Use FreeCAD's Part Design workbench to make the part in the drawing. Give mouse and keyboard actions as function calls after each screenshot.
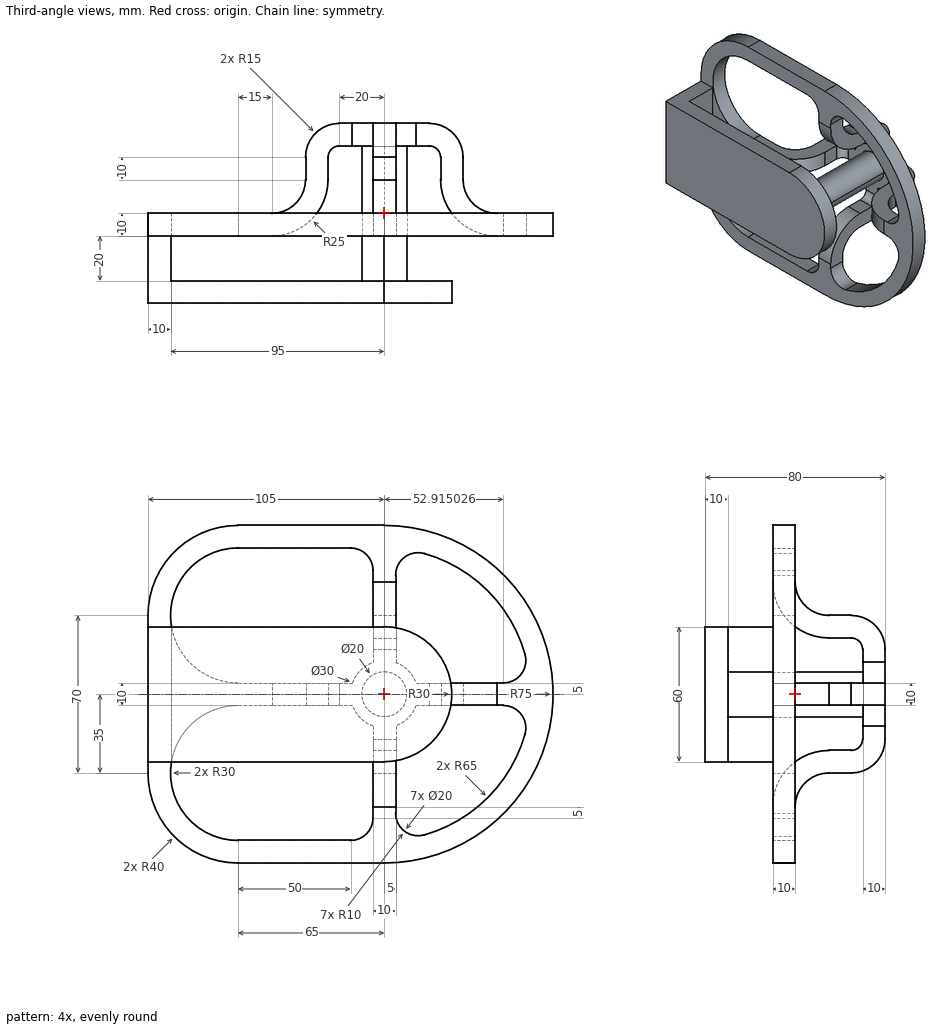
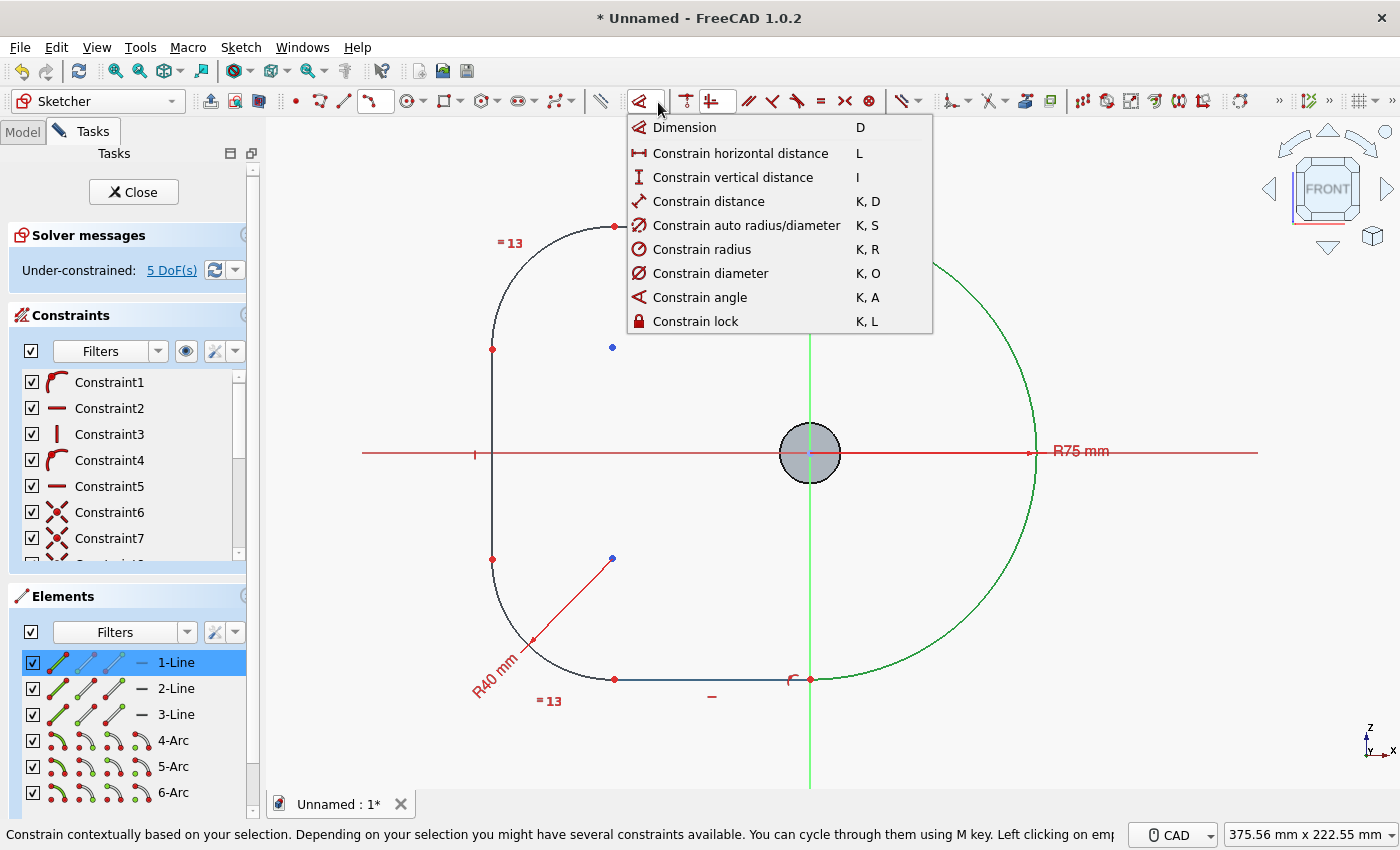
click(780, 153)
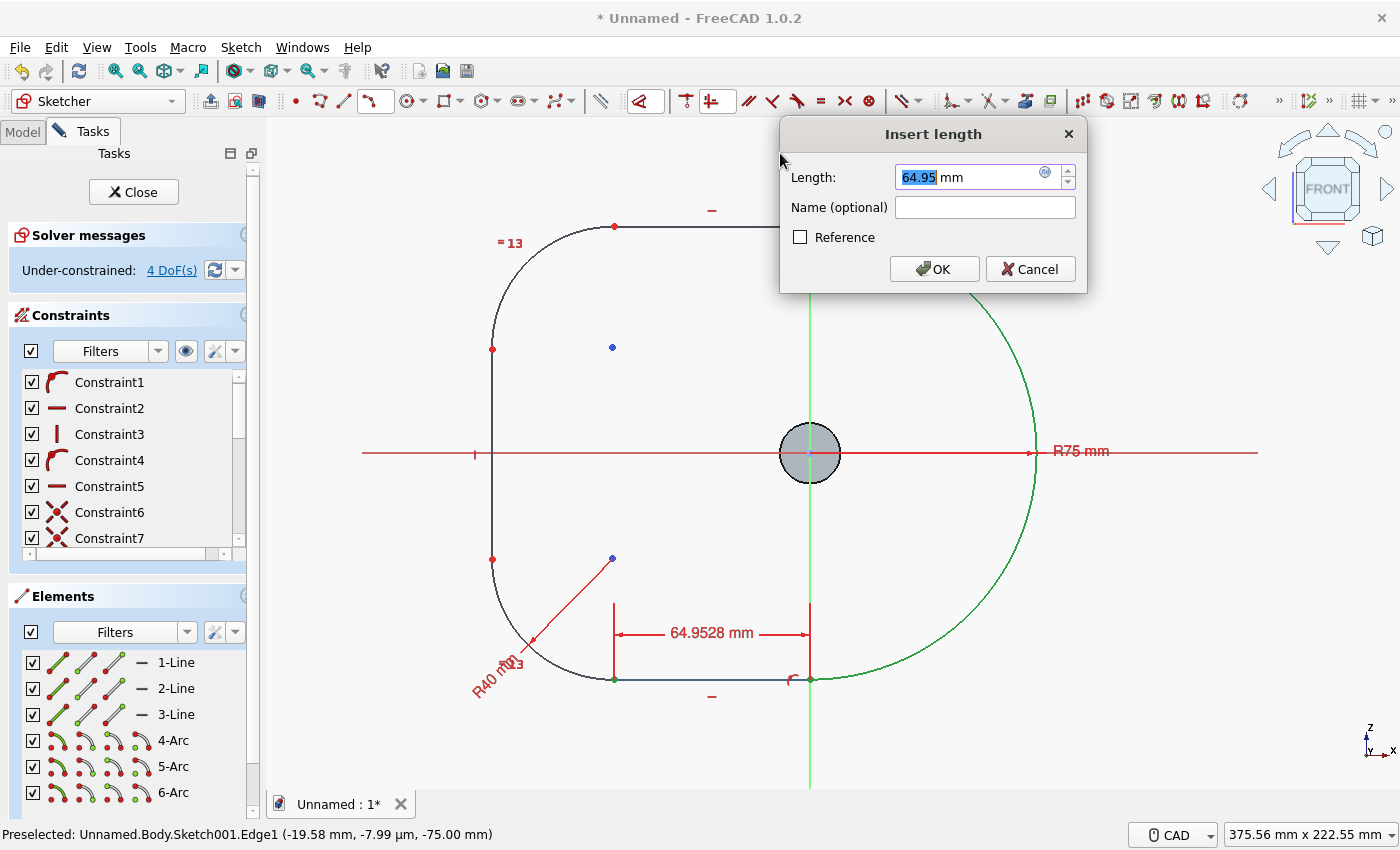
text(65)
key(Return)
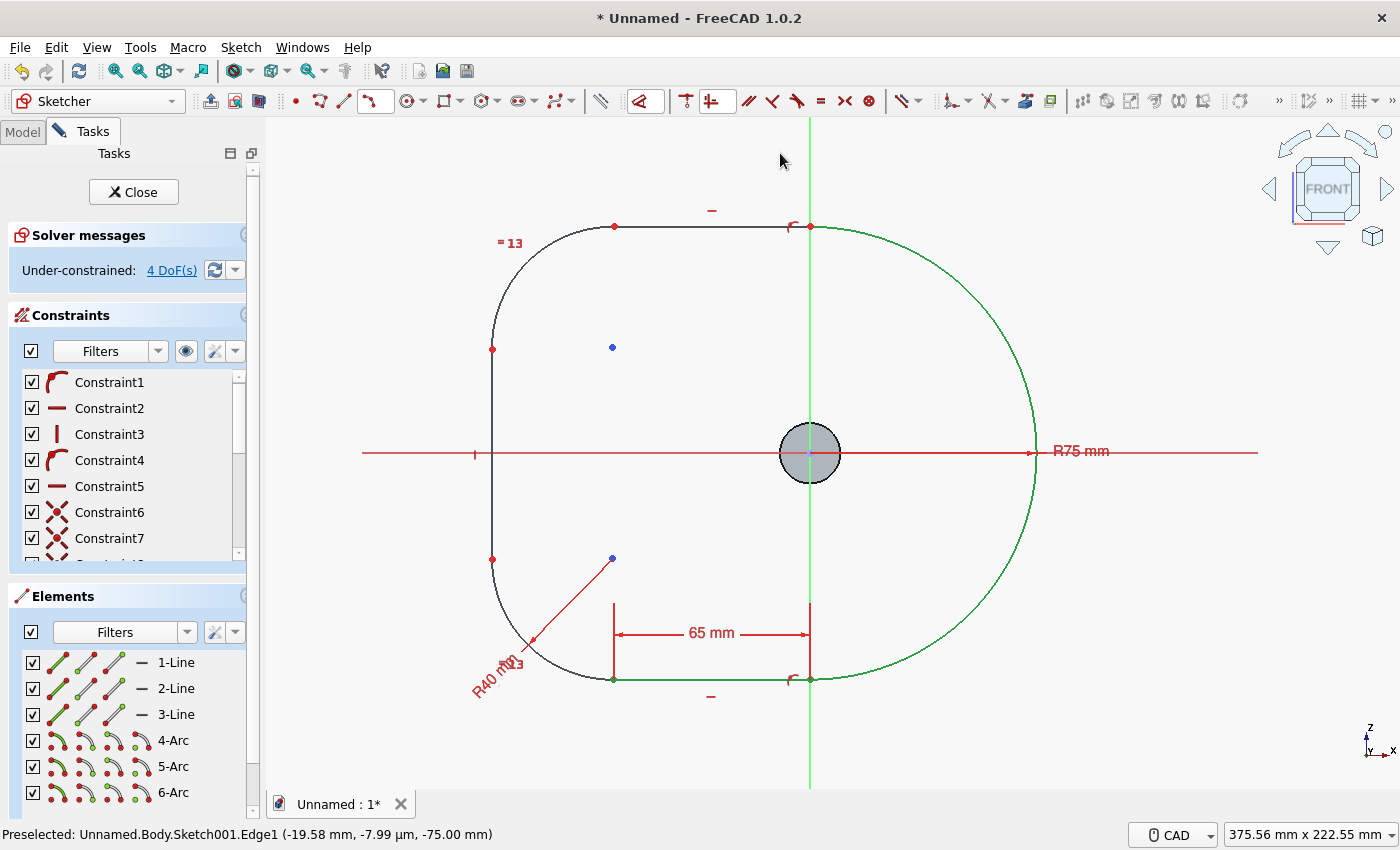
click(492, 497)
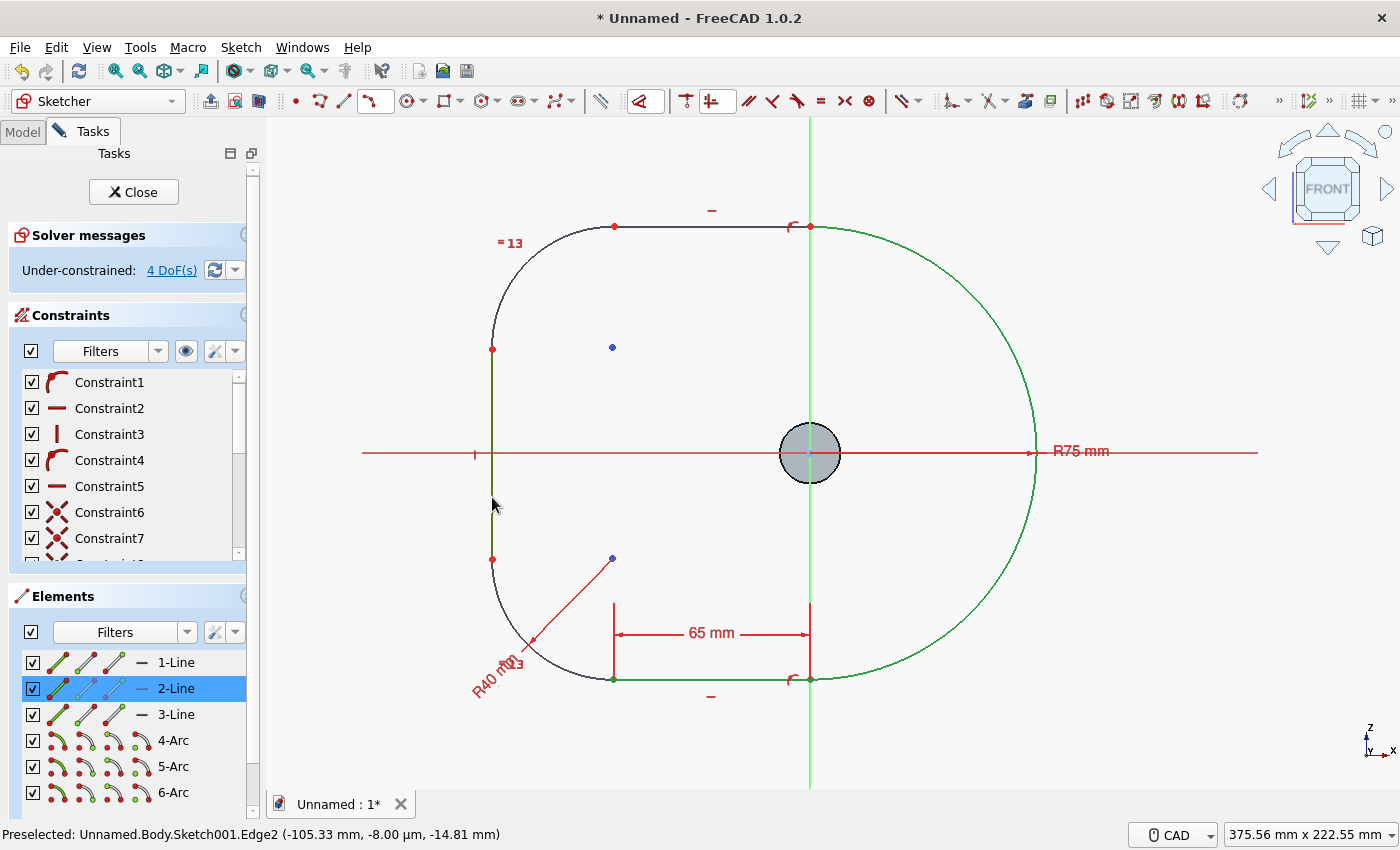
click(658, 102)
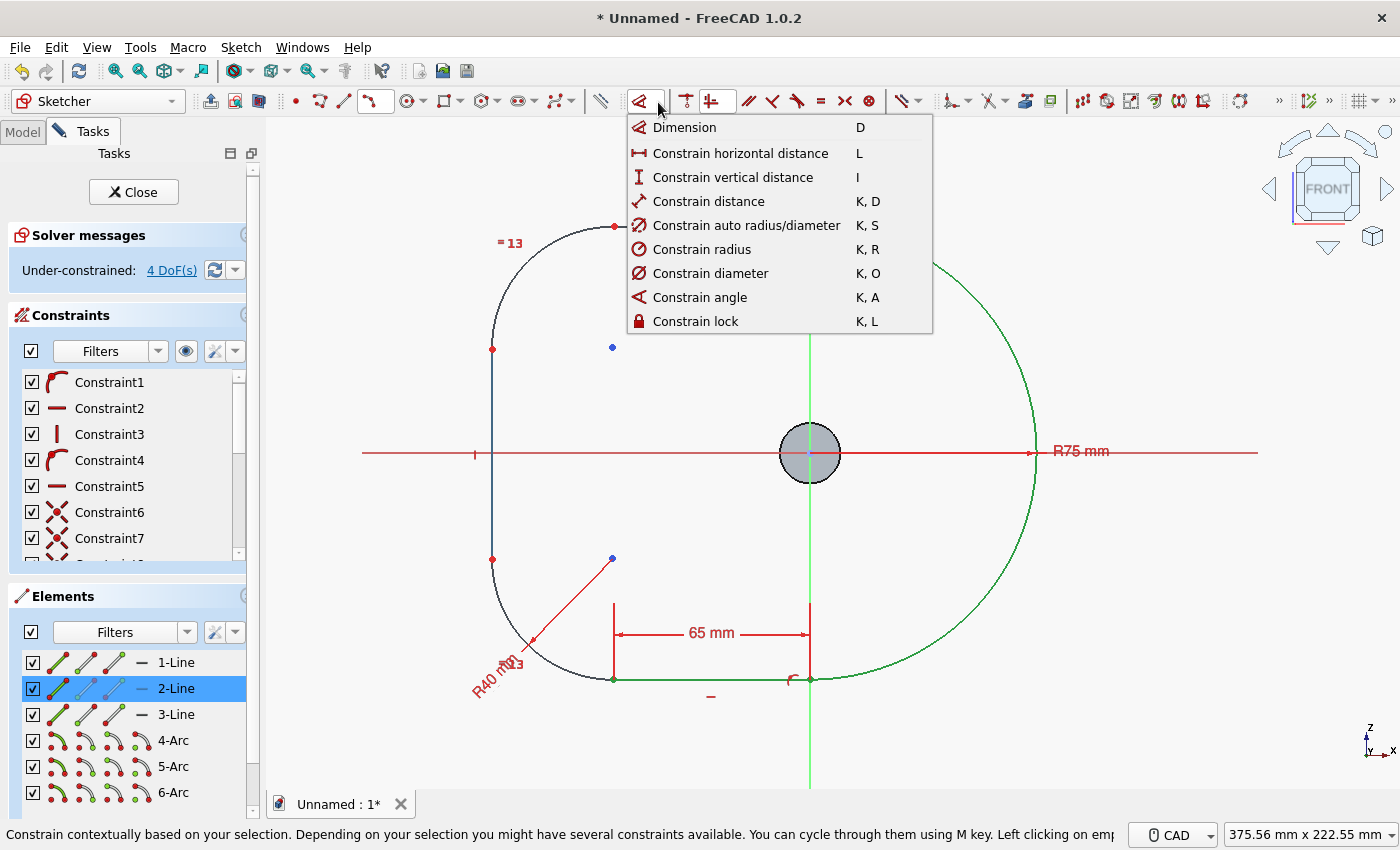
click(780, 177)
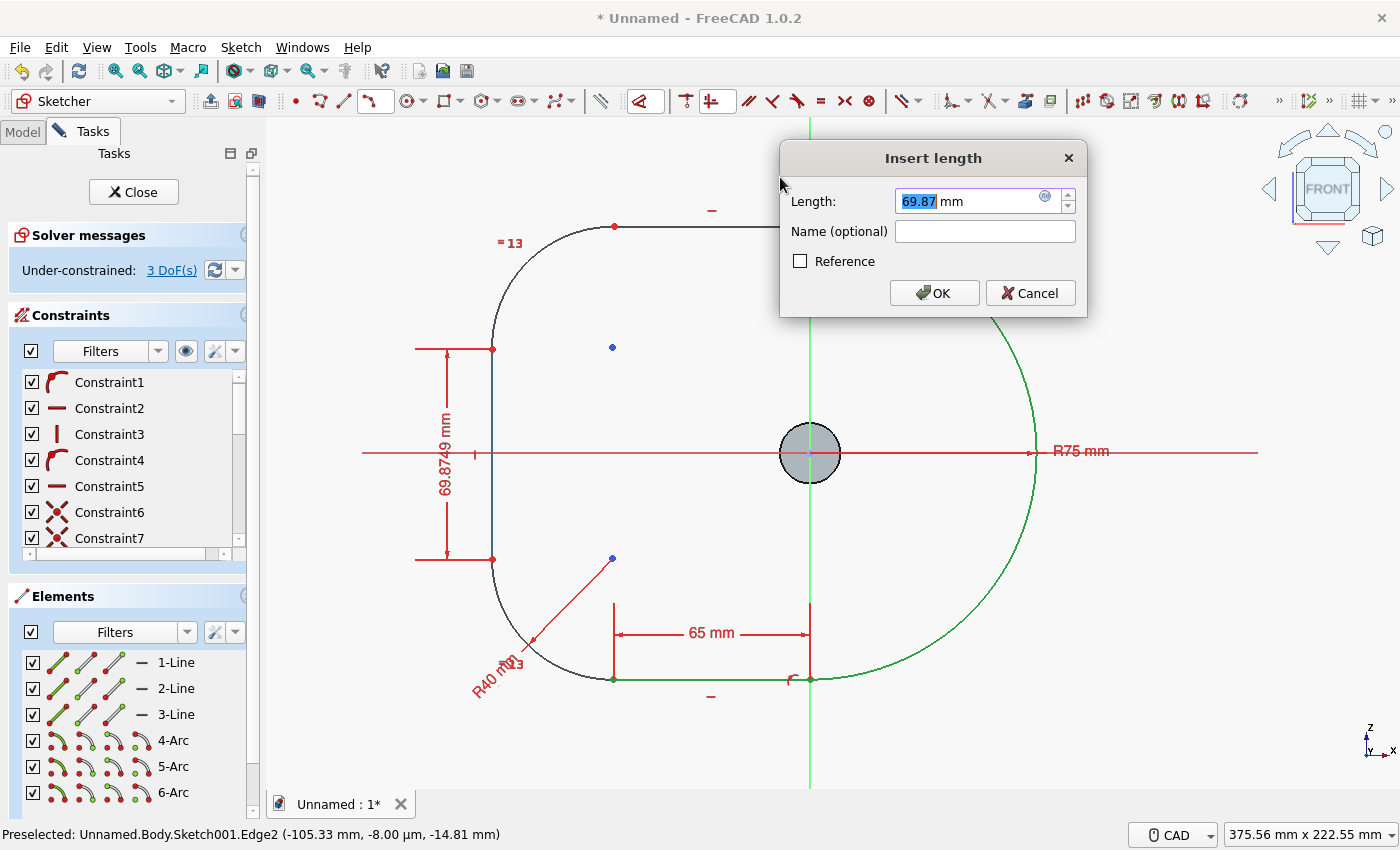
text(70)
key(Return)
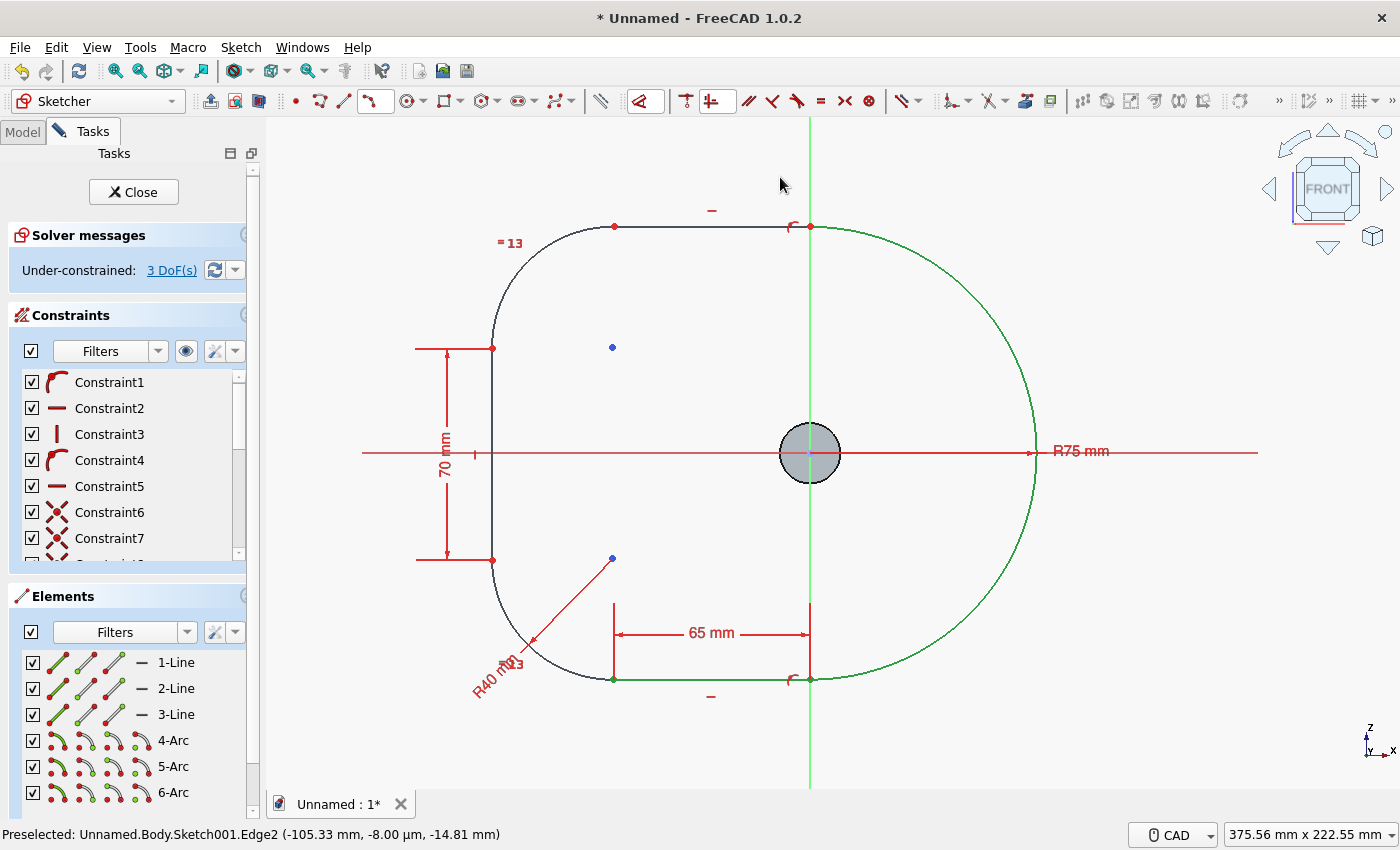
click(673, 227)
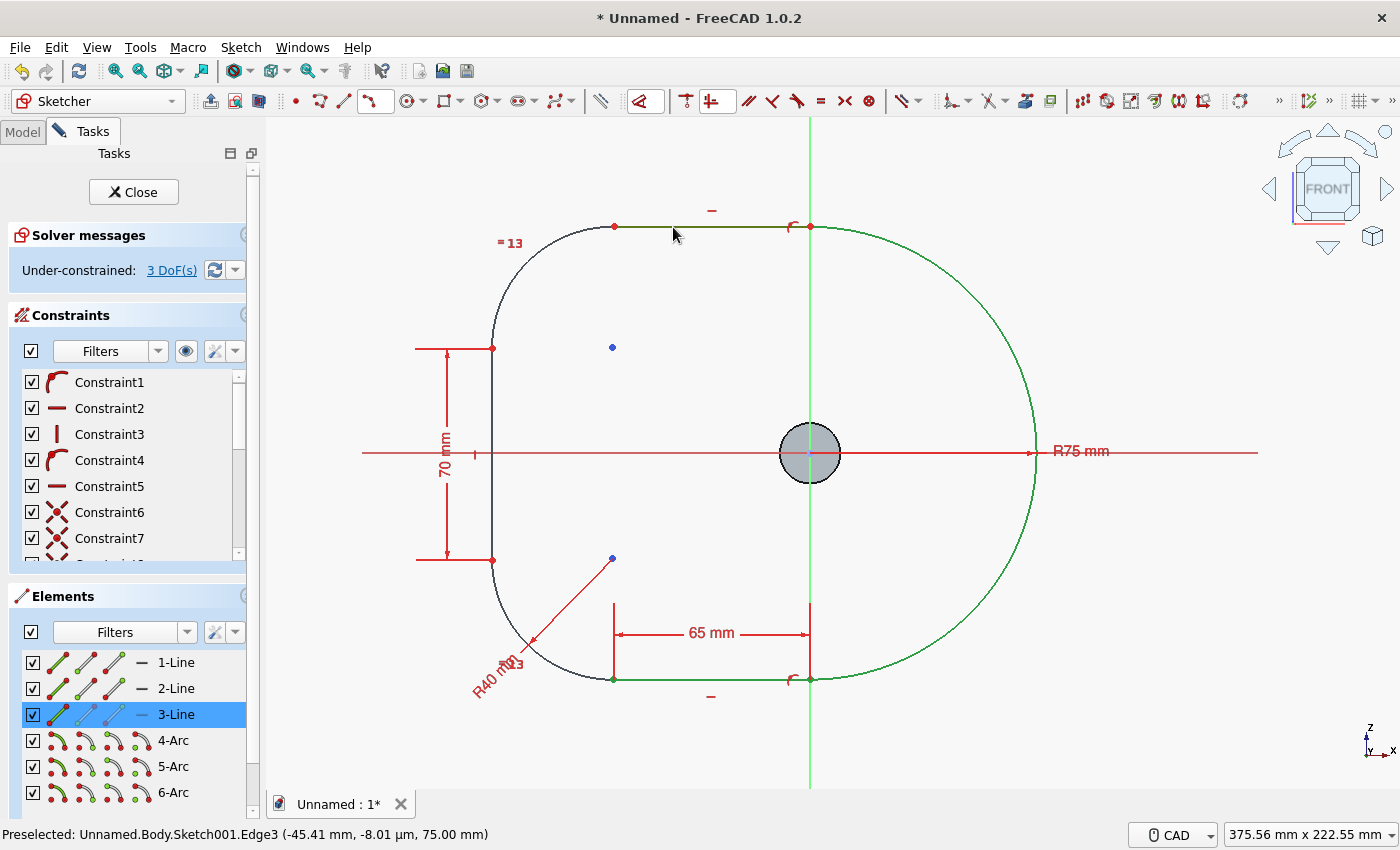
key(l)